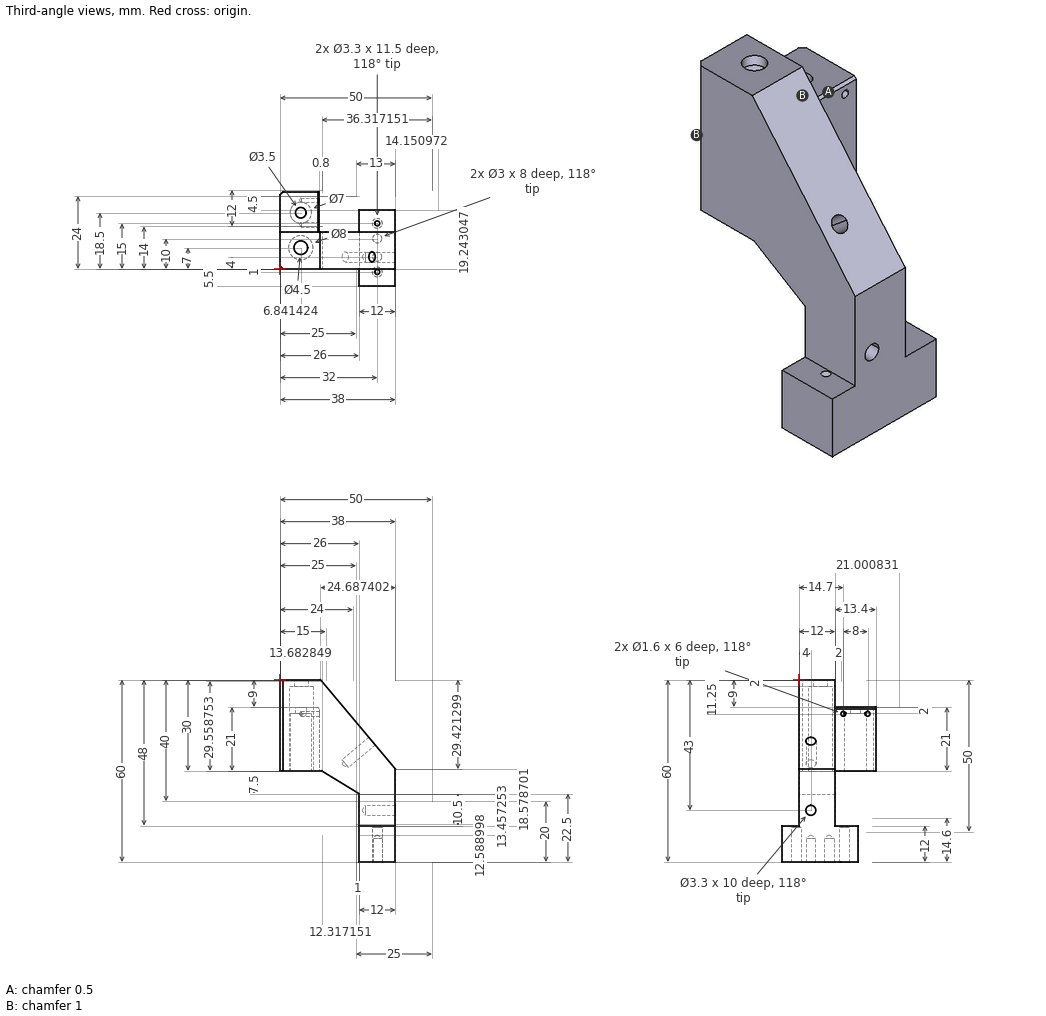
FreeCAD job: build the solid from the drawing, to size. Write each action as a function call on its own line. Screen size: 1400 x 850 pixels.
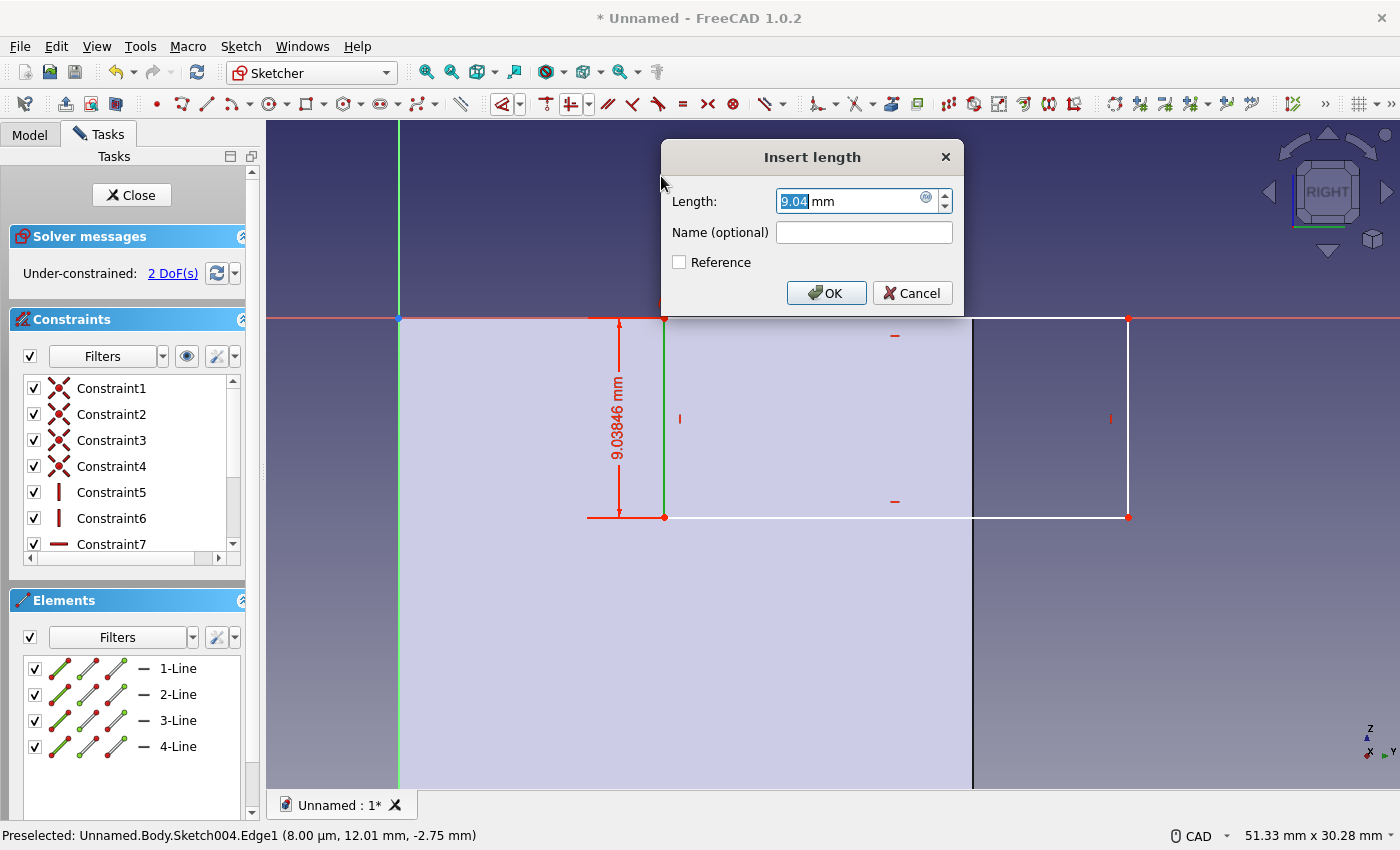
text(9)
key(Return)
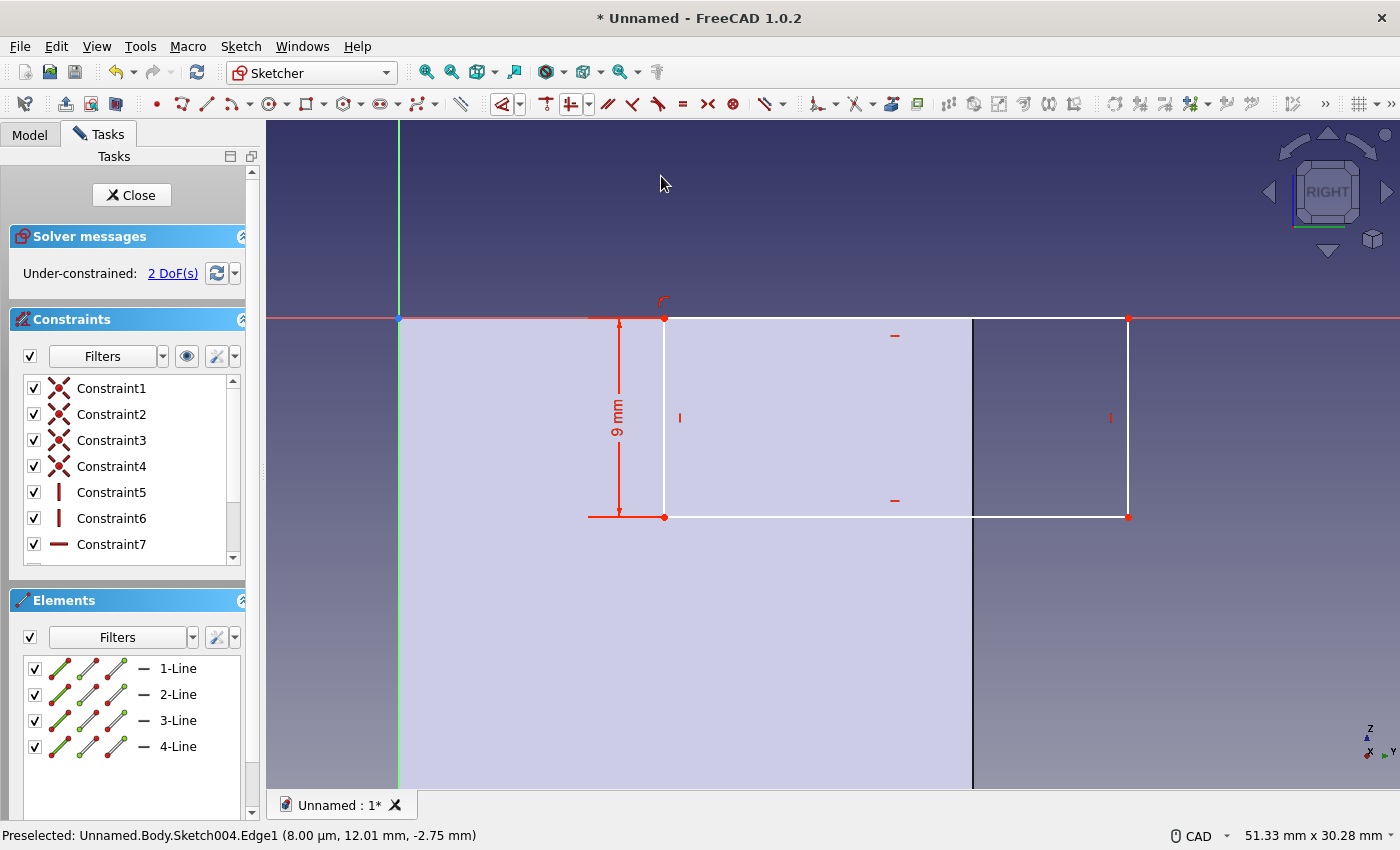
click(664, 318)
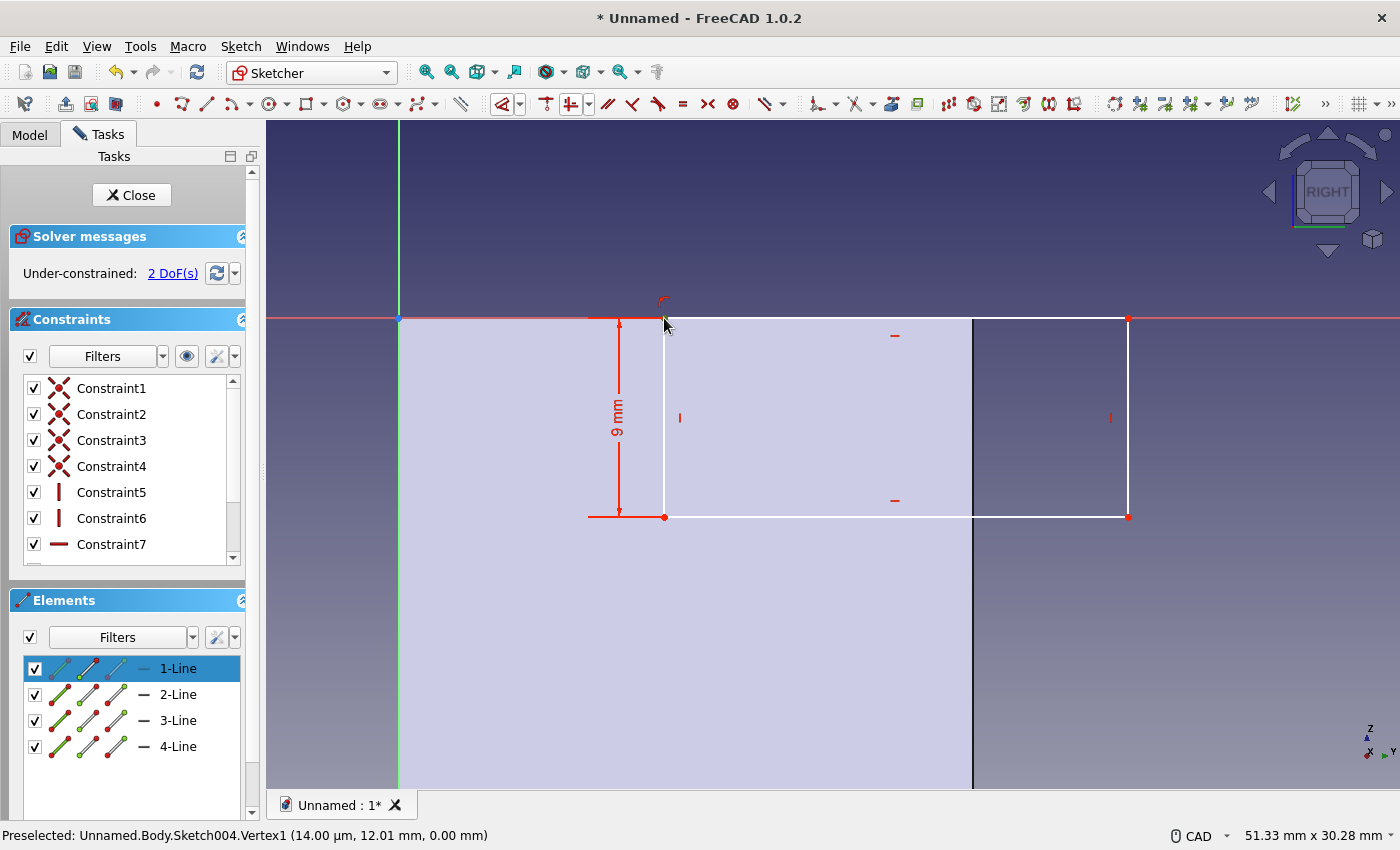
key(l)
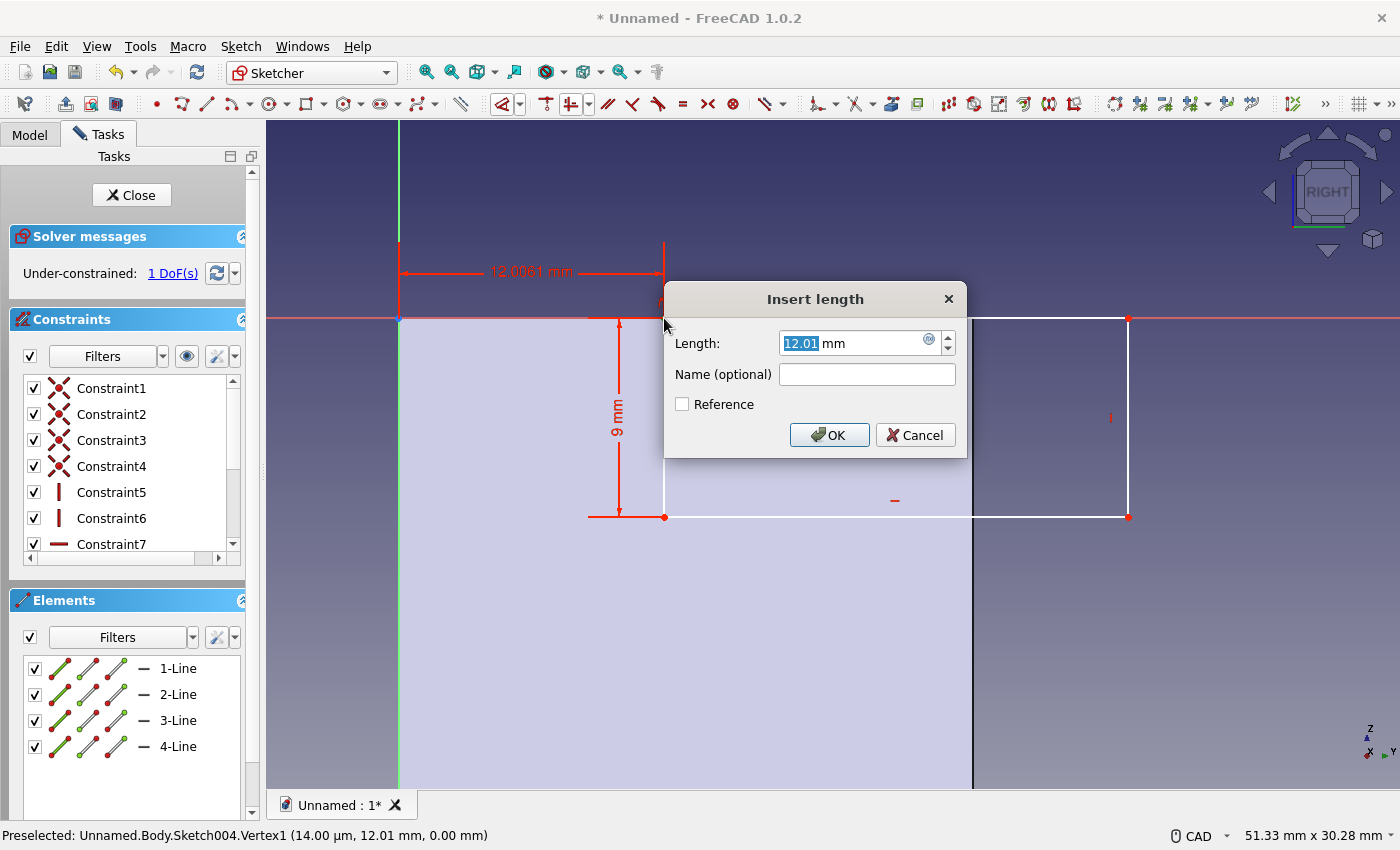
text(12)
key(Return)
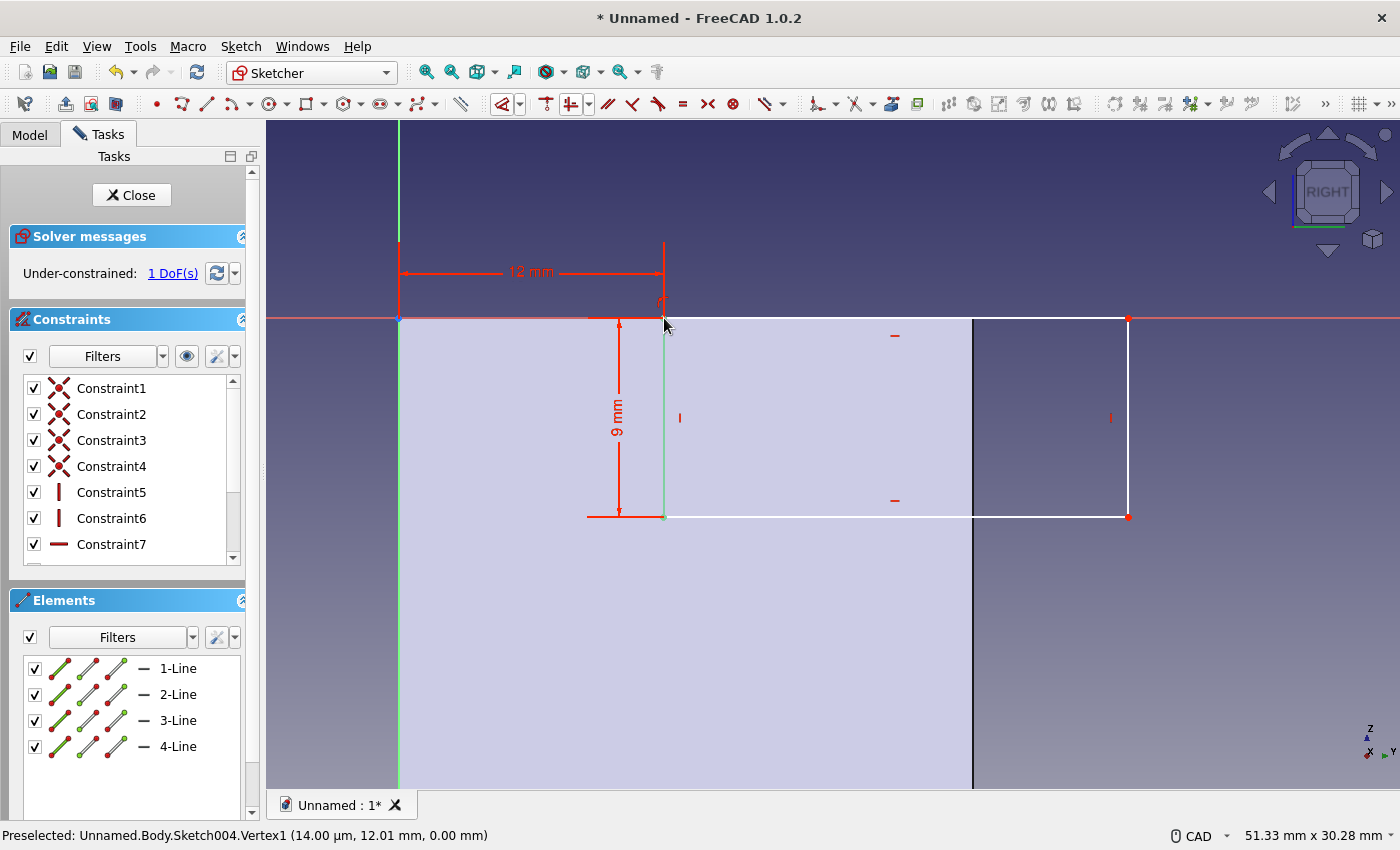
click(803, 517)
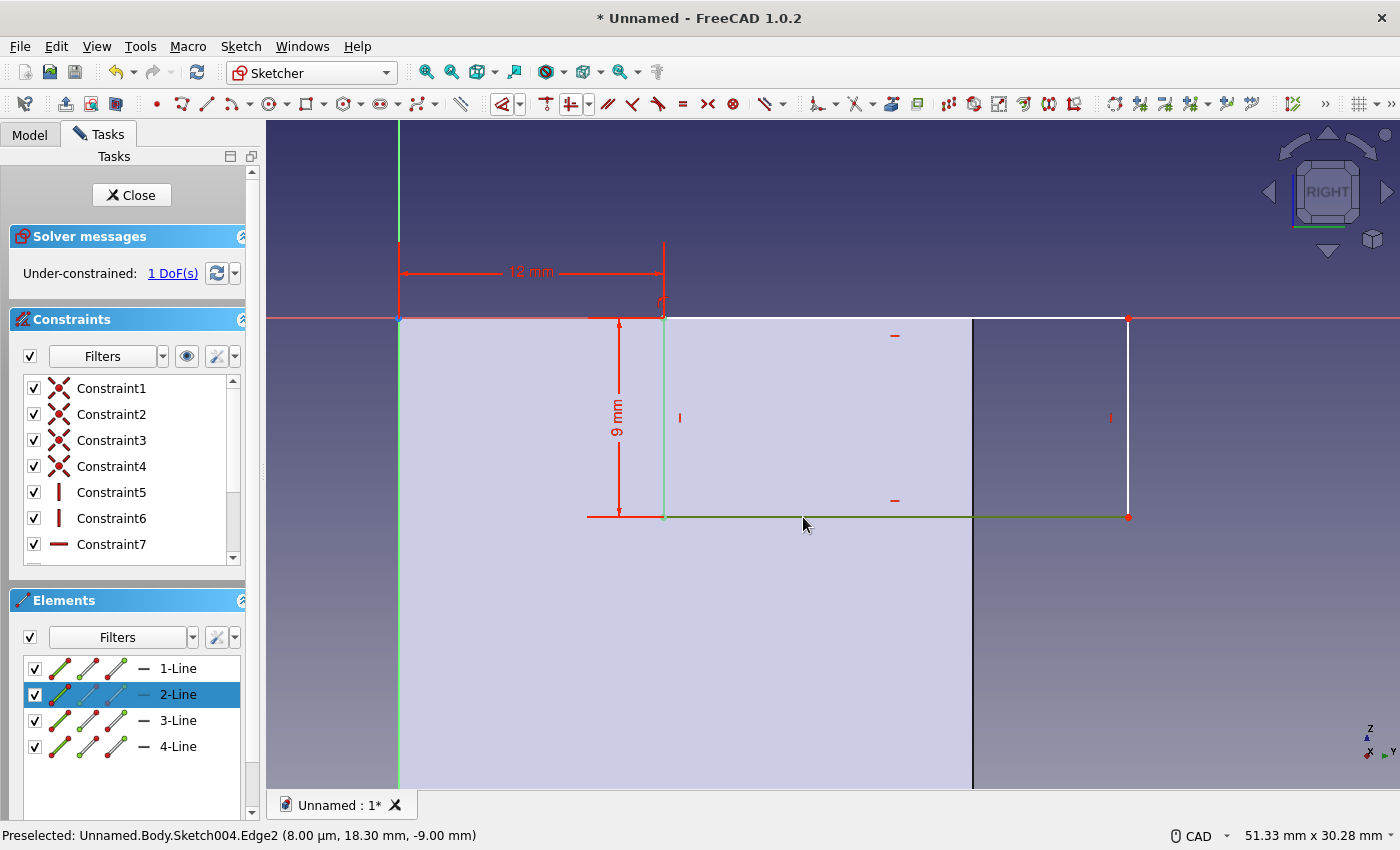
click(520, 104)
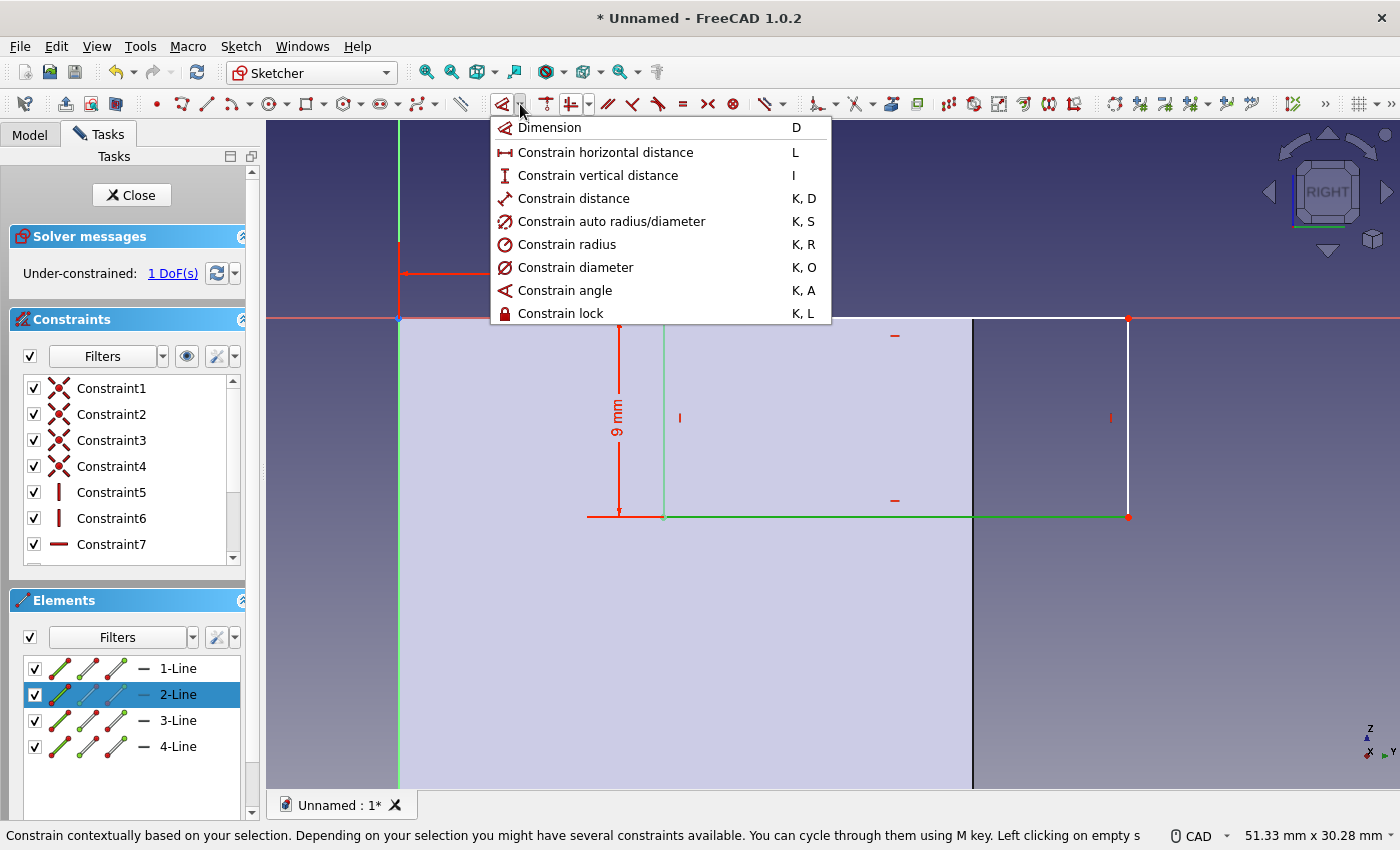
click(661, 152)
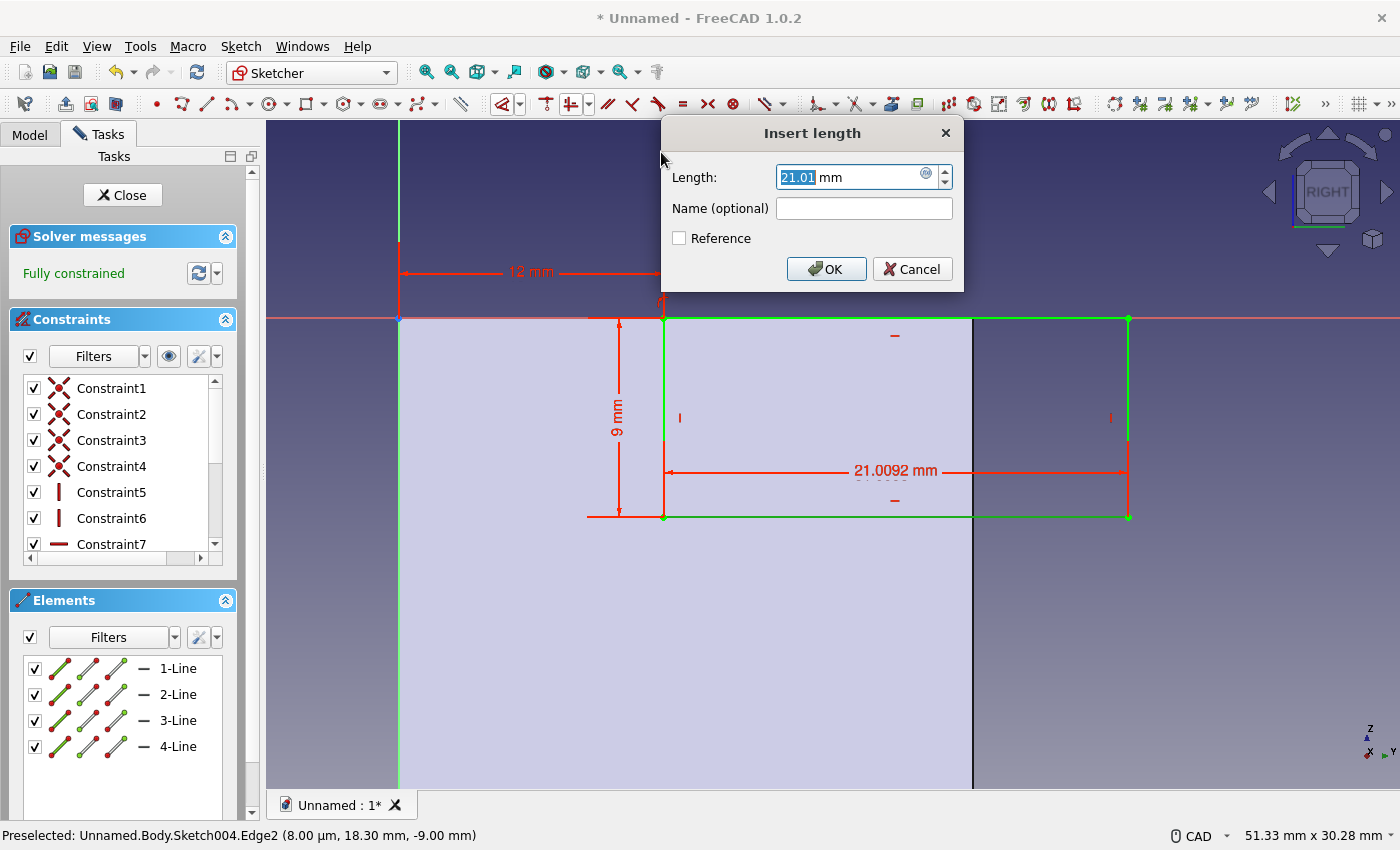
text(21.000831)
key(Return)